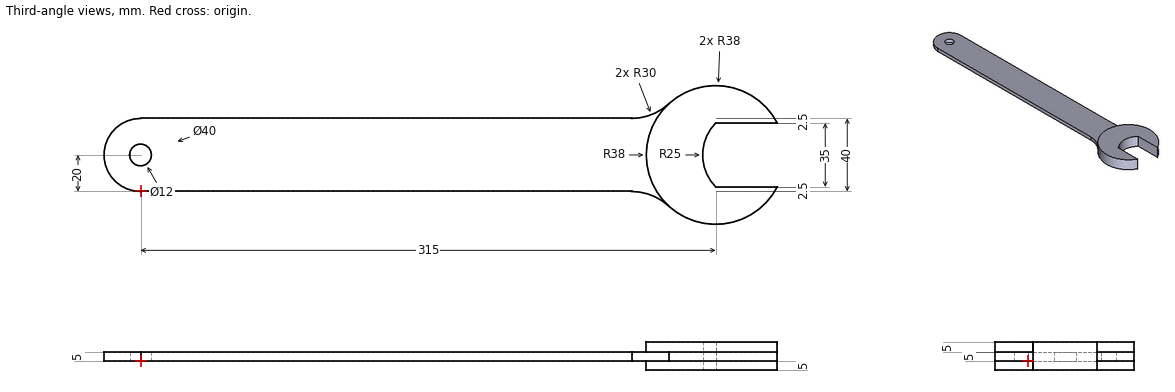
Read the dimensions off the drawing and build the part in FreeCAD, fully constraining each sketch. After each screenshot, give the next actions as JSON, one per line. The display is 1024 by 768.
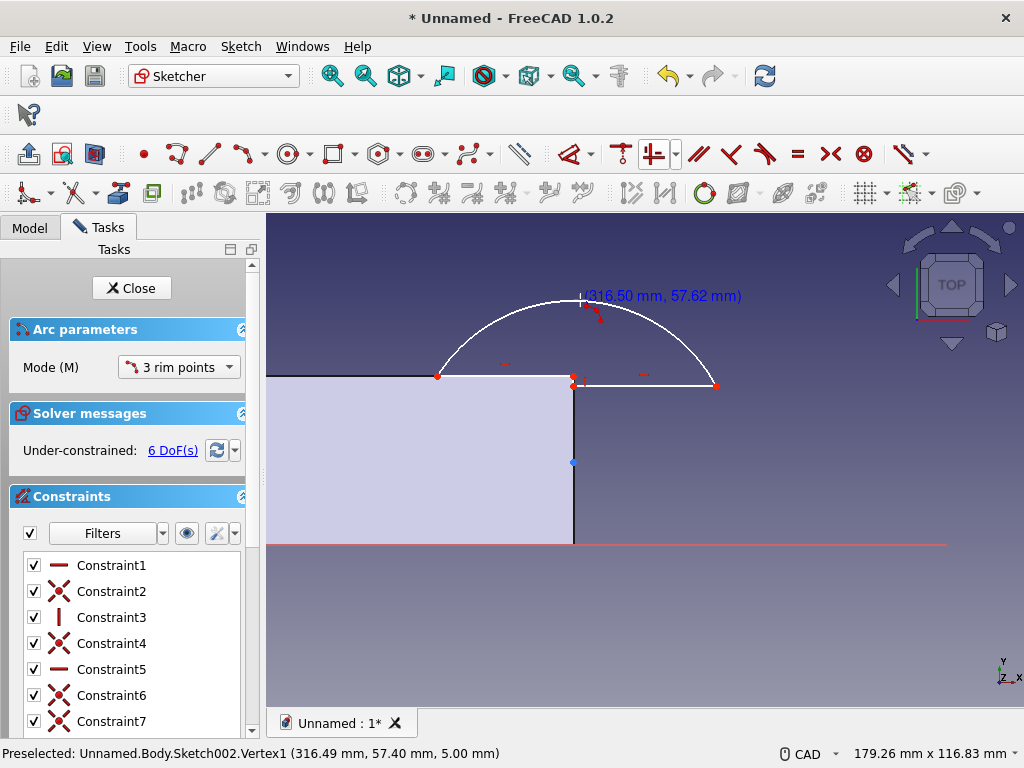
{"action": "left_click", "coordinate": [177, 154]}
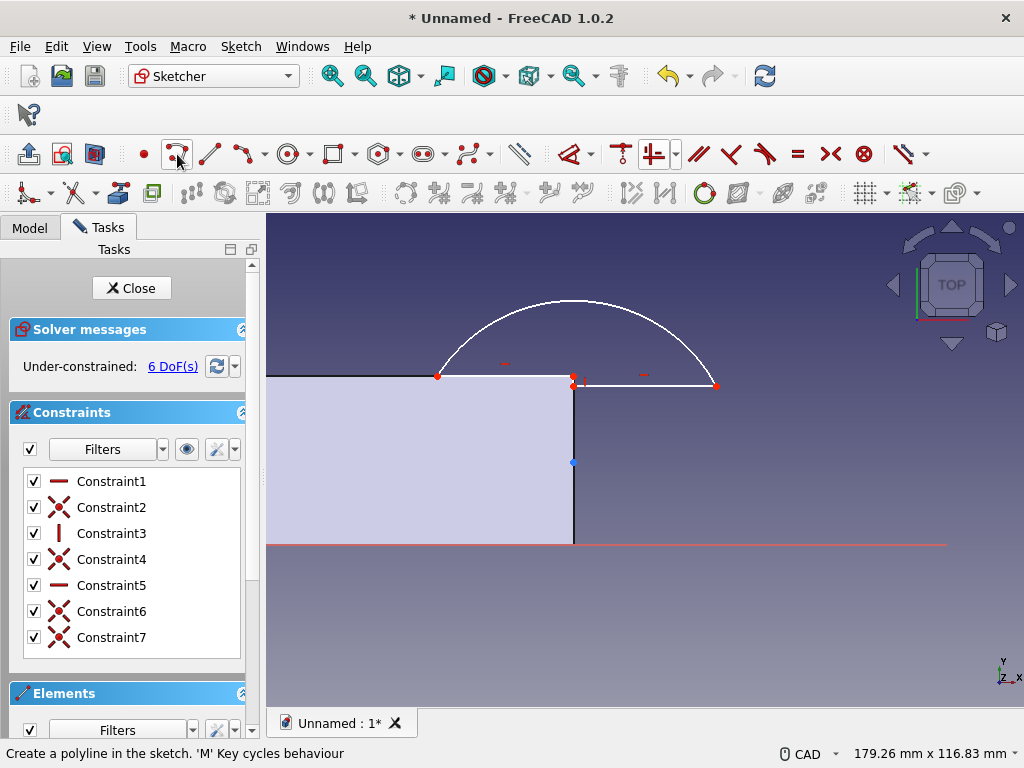
{"action": "scroll", "coordinate": [716, 534], "scroll_direction": "up", "scroll_amount": 3}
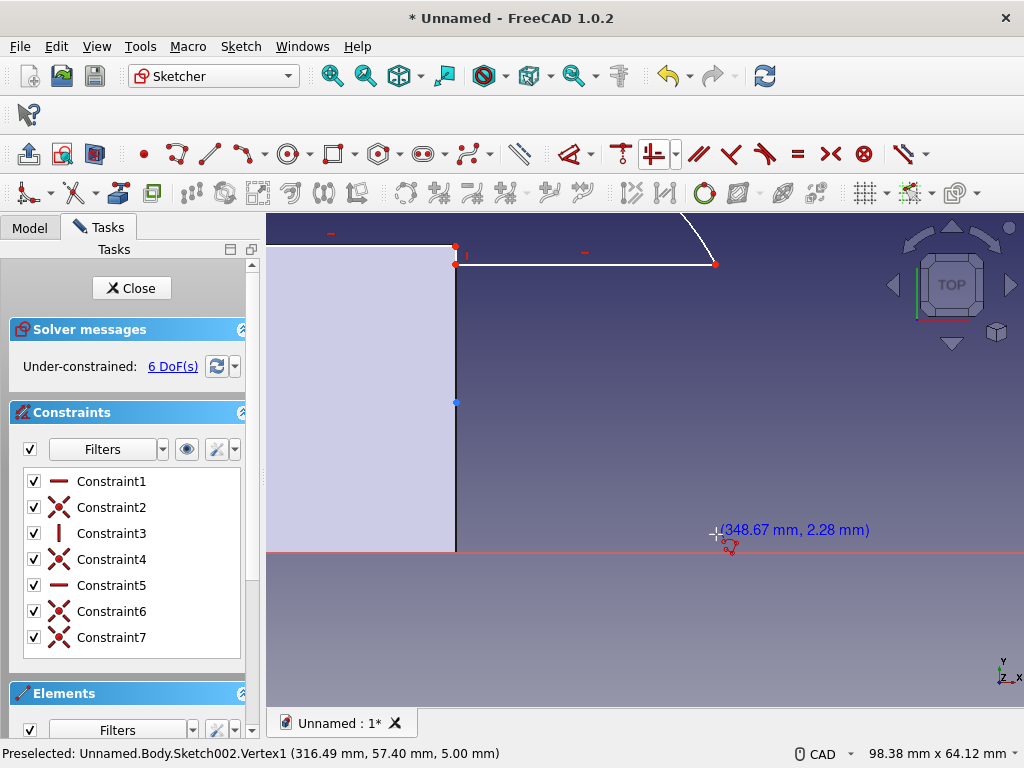
{"action": "left_click", "coordinate": [716, 534]}
{"action": "left_click", "coordinate": [456, 534]}
{"action": "left_click", "coordinate": [456, 553]}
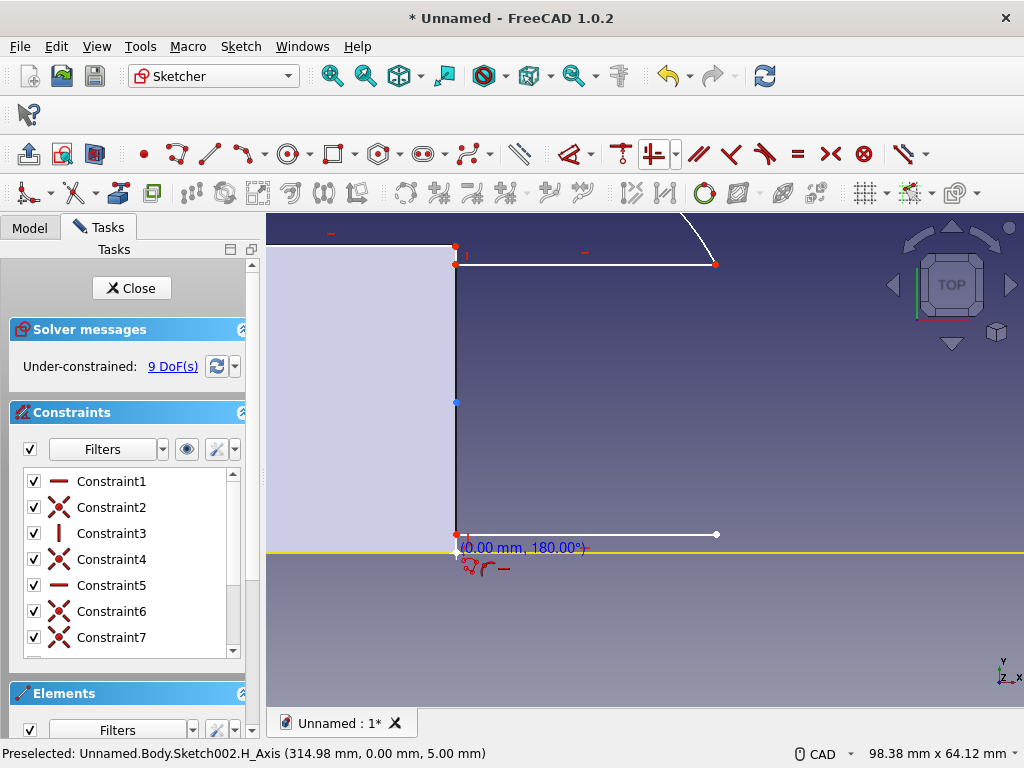
{"action": "scroll", "coordinate": [716, 534], "scroll_direction": "down", "scroll_amount": 3}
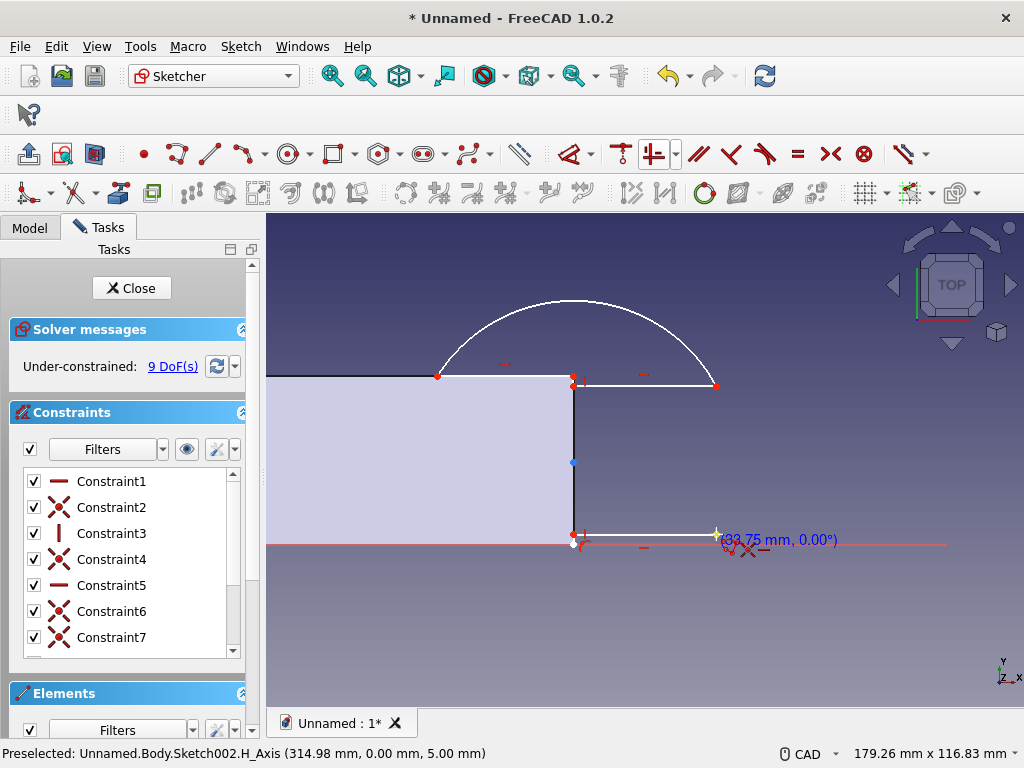
{"action": "left_click", "coordinate": [437, 536]}
{"action": "right_click", "coordinate": [437, 536]}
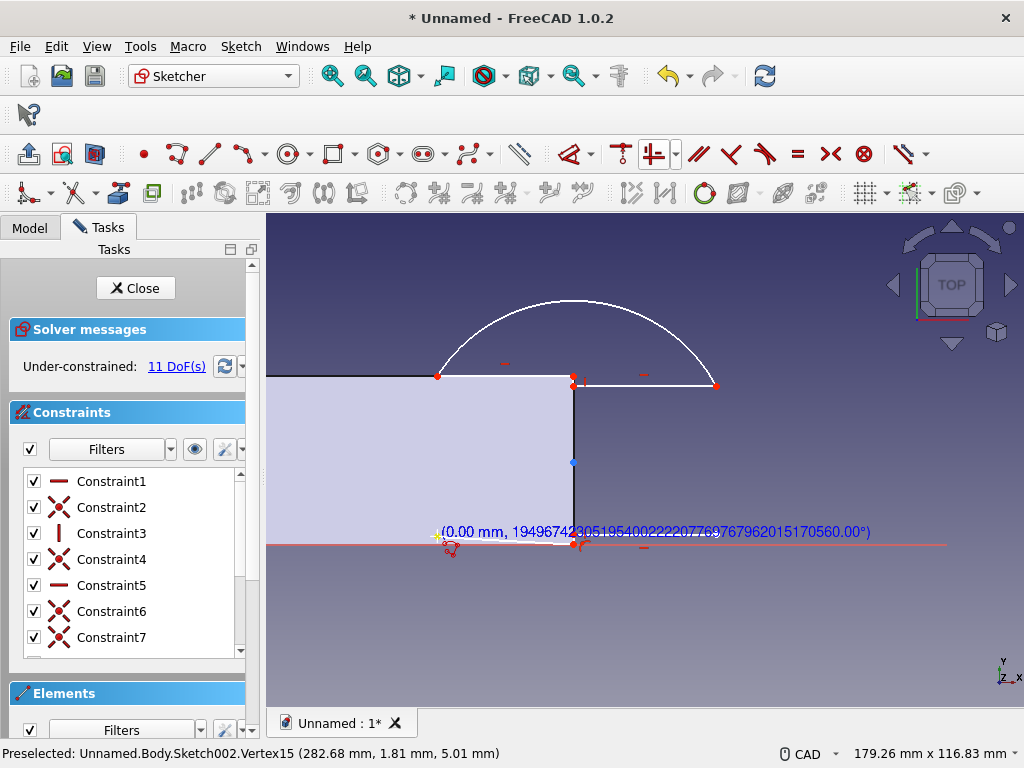
{"action": "left_click", "coordinate": [242, 154]}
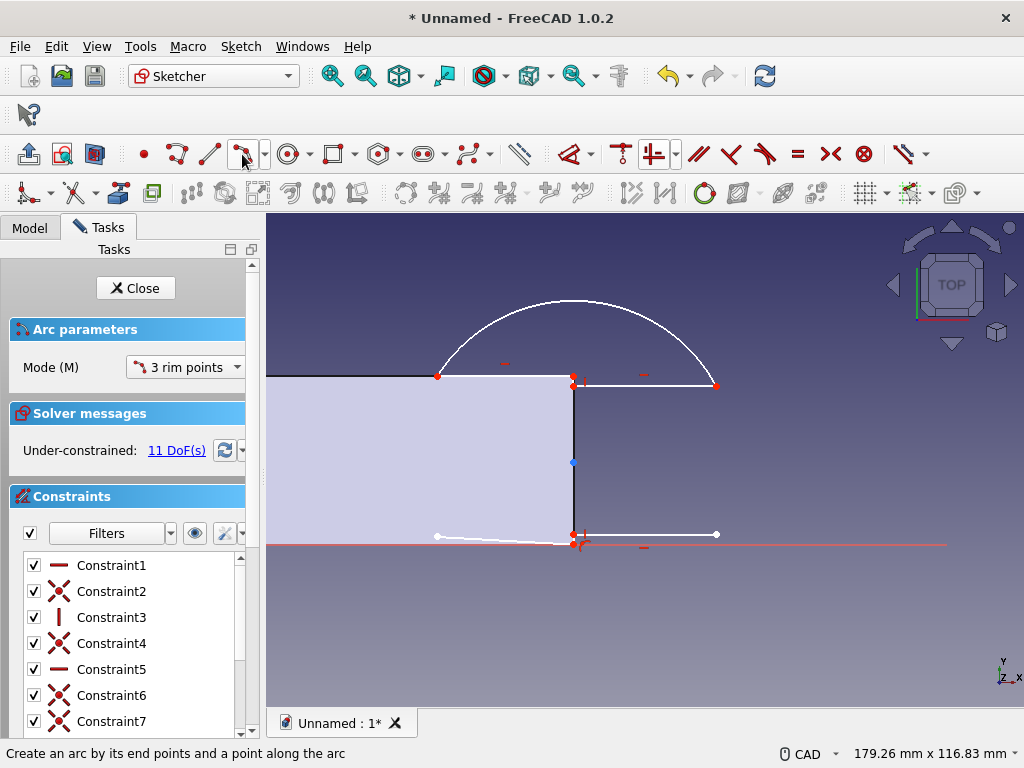
{"action": "left_click", "coordinate": [437, 537]}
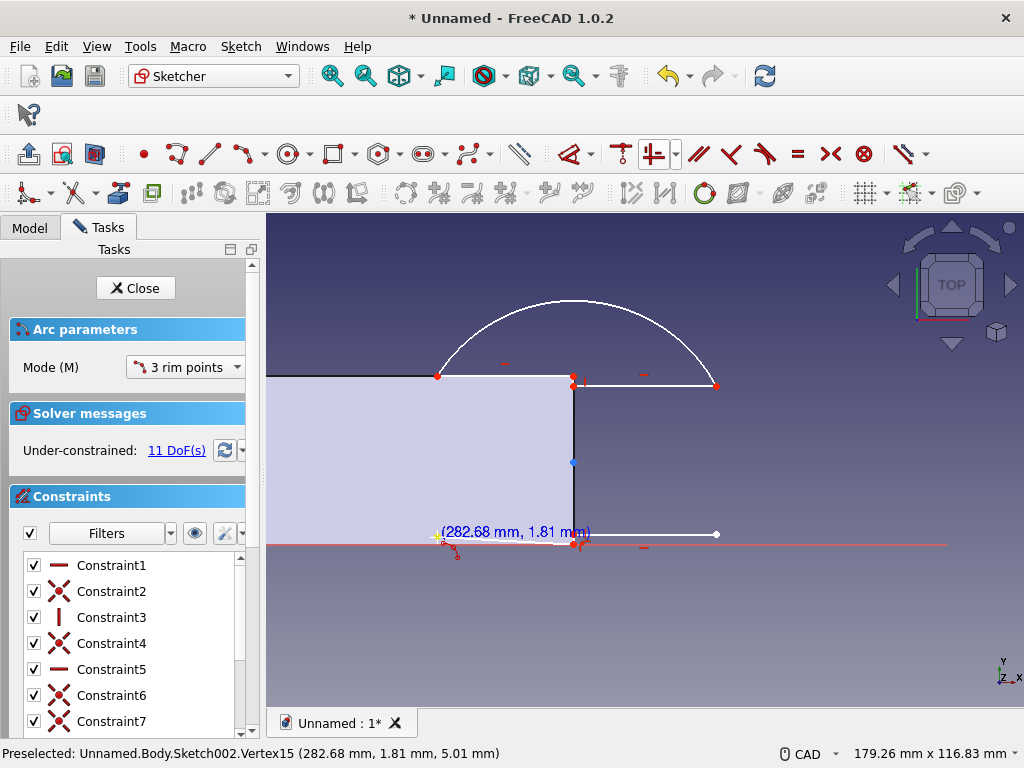
{"action": "scroll", "coordinate": [716, 534], "scroll_direction": "up", "scroll_amount": 3}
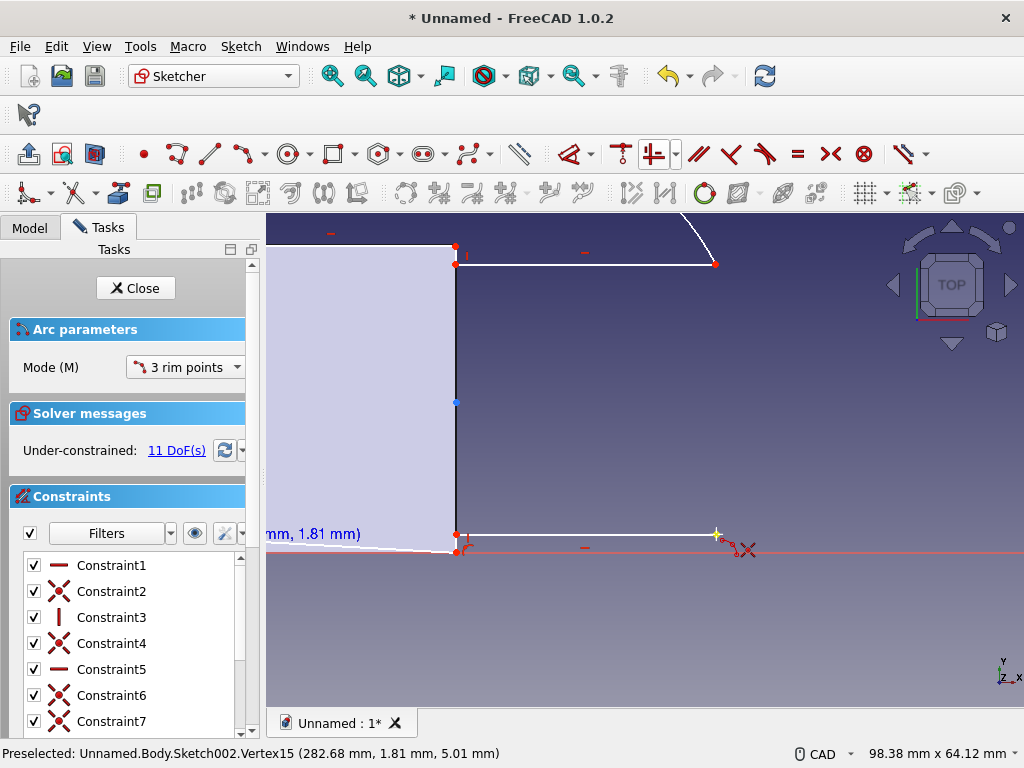
{"action": "left_click", "coordinate": [716, 535]}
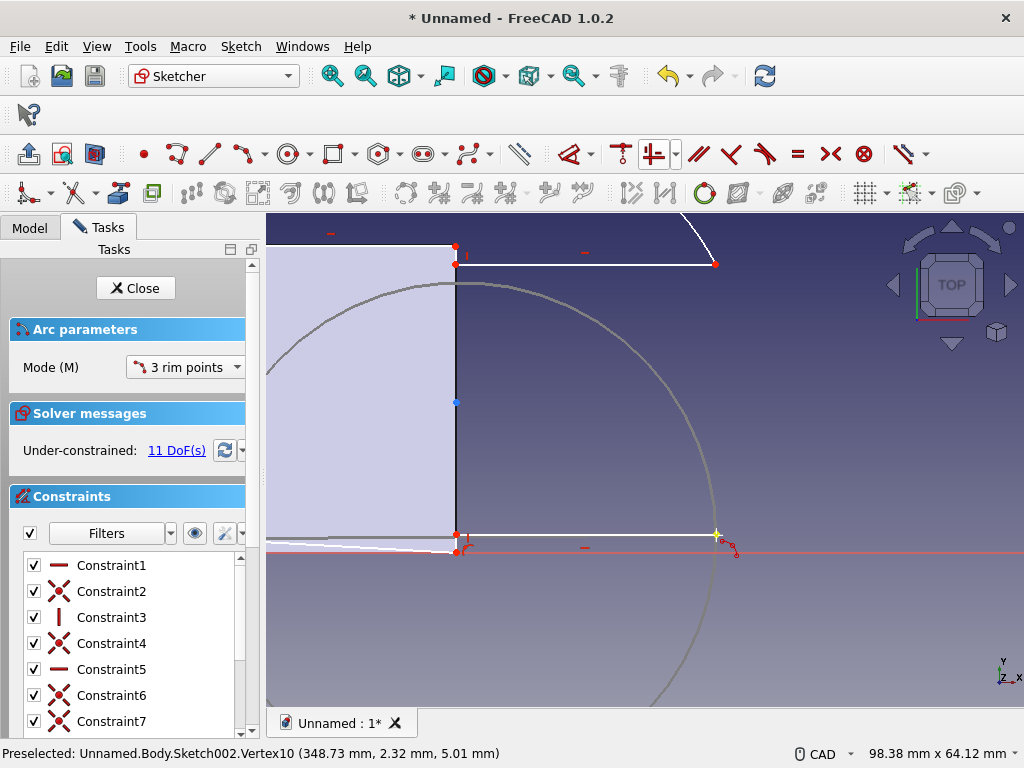
{"action": "scroll", "coordinate": [716, 534], "scroll_direction": "down", "scroll_amount": 3}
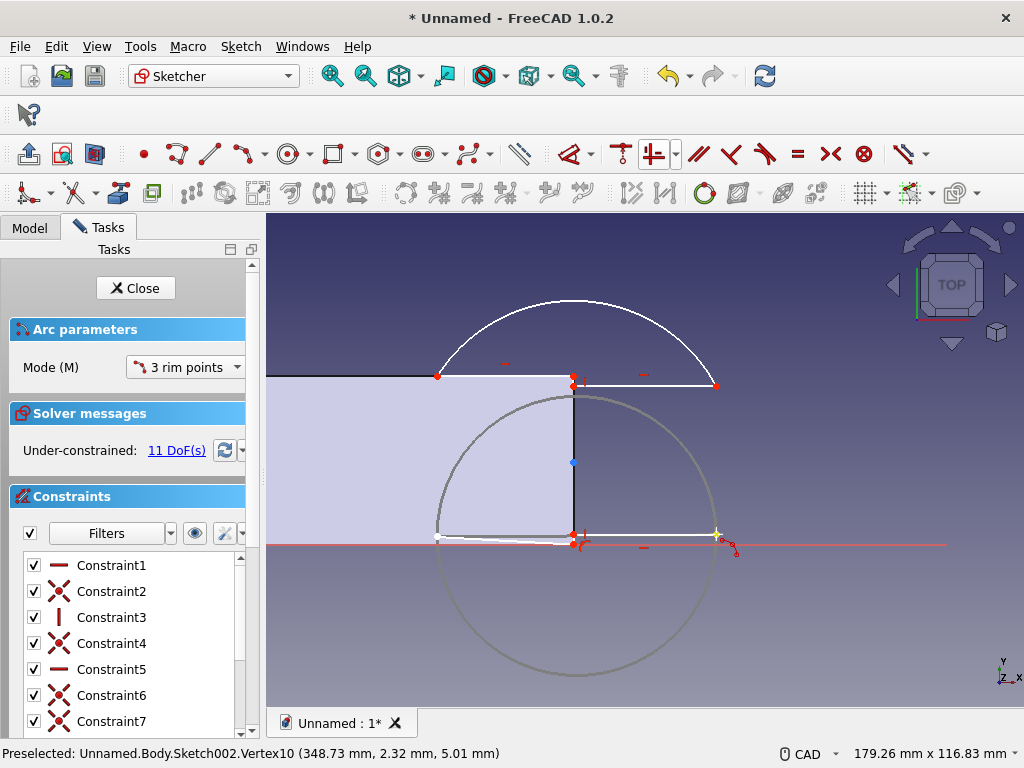
{"action": "left_click", "coordinate": [580, 621]}
{"action": "key", "text": "Escape"}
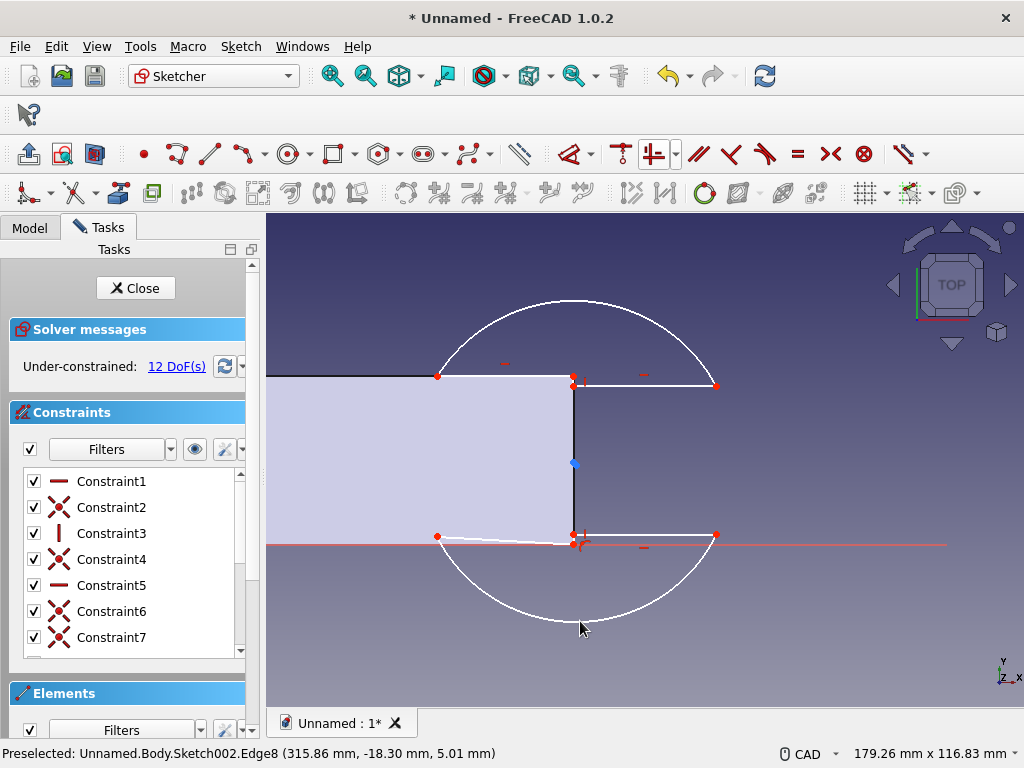
{"action": "left_click", "coordinate": [533, 542]}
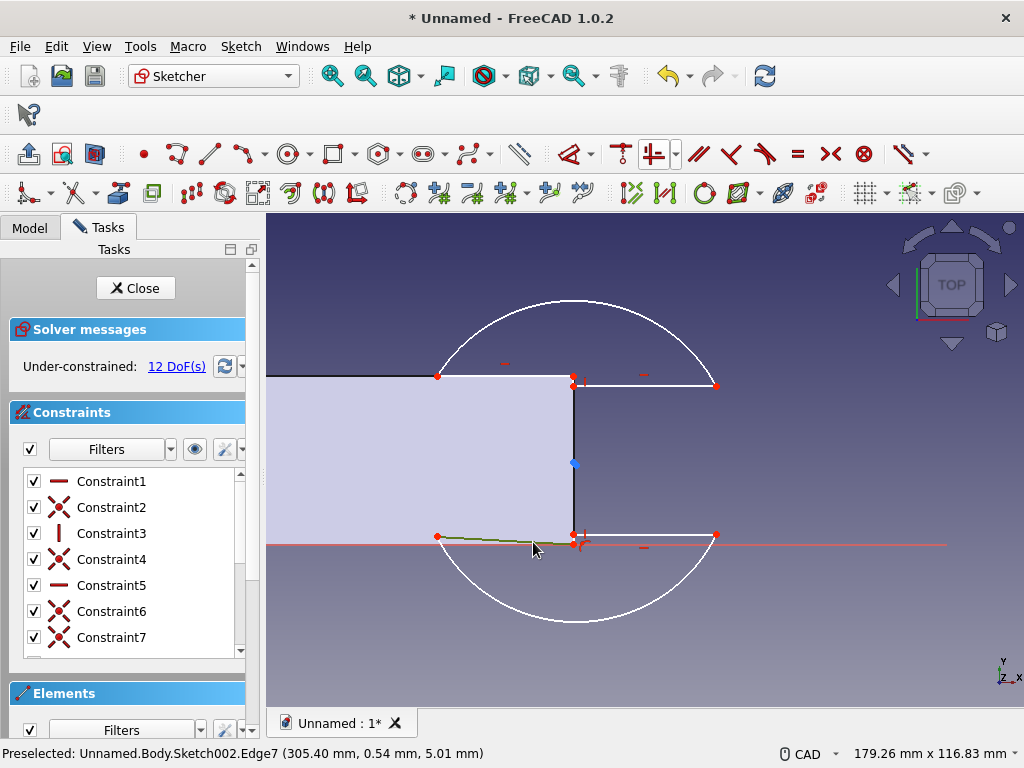
{"action": "left_click", "coordinate": [676, 154]}